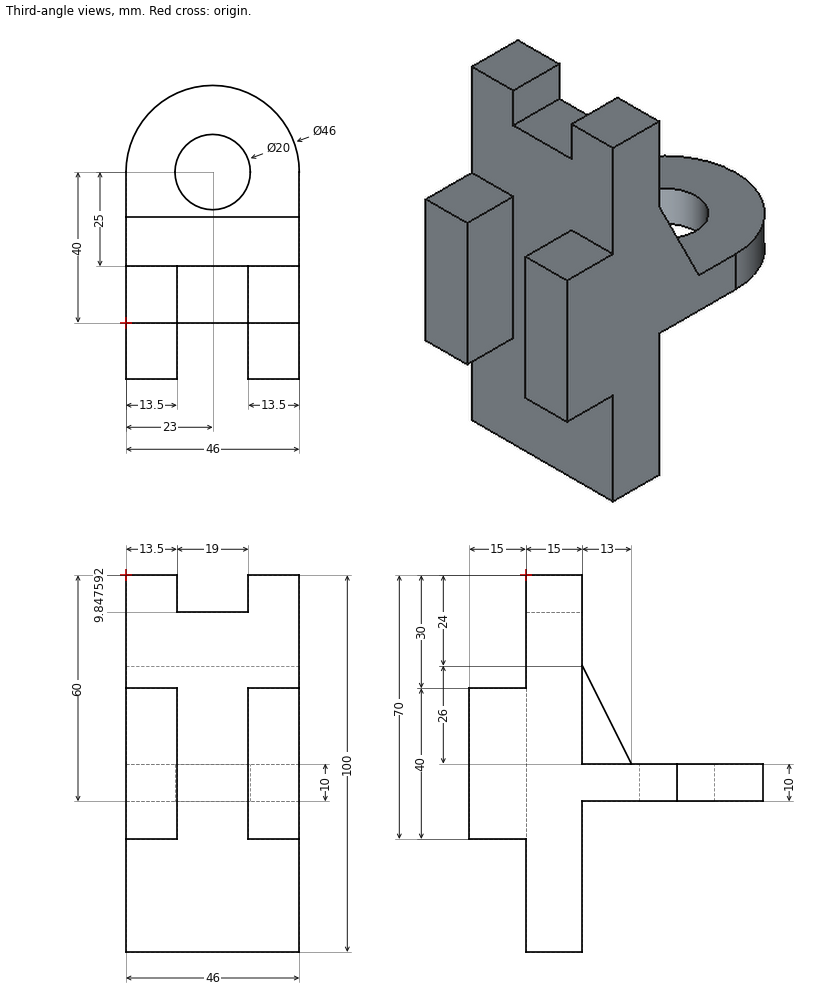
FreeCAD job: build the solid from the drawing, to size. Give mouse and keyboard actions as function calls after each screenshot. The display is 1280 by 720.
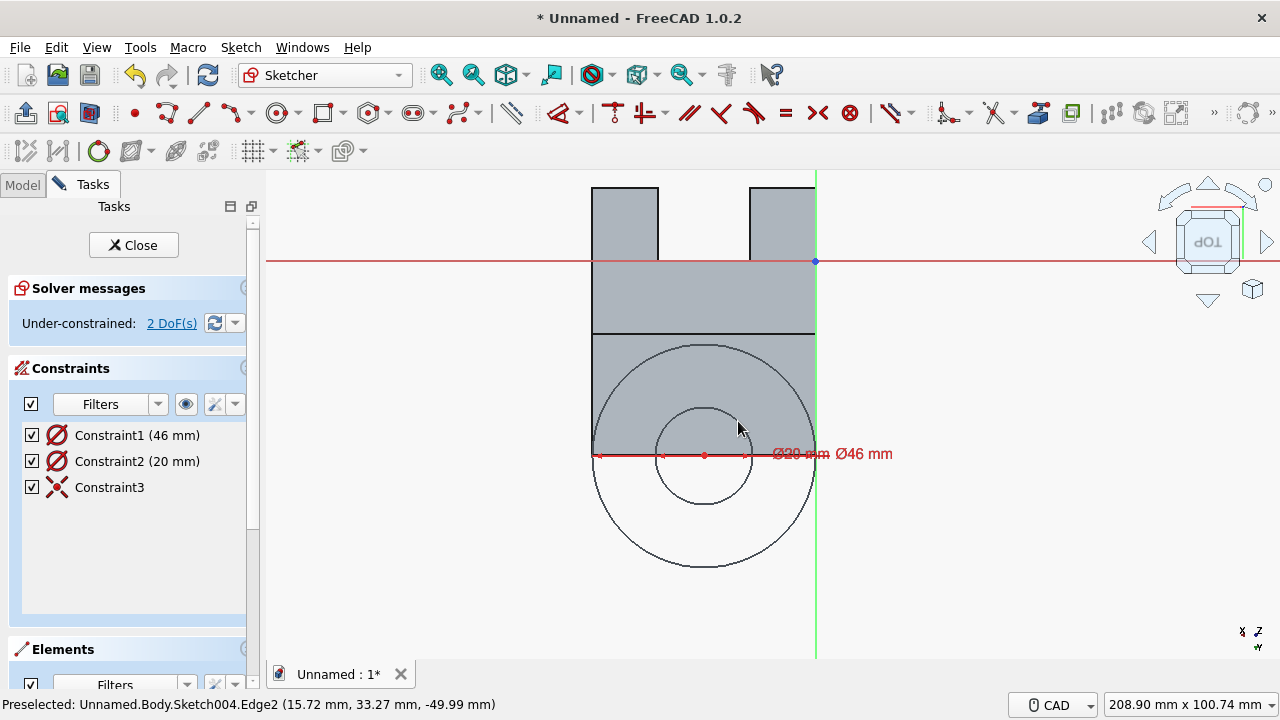
click(558, 114)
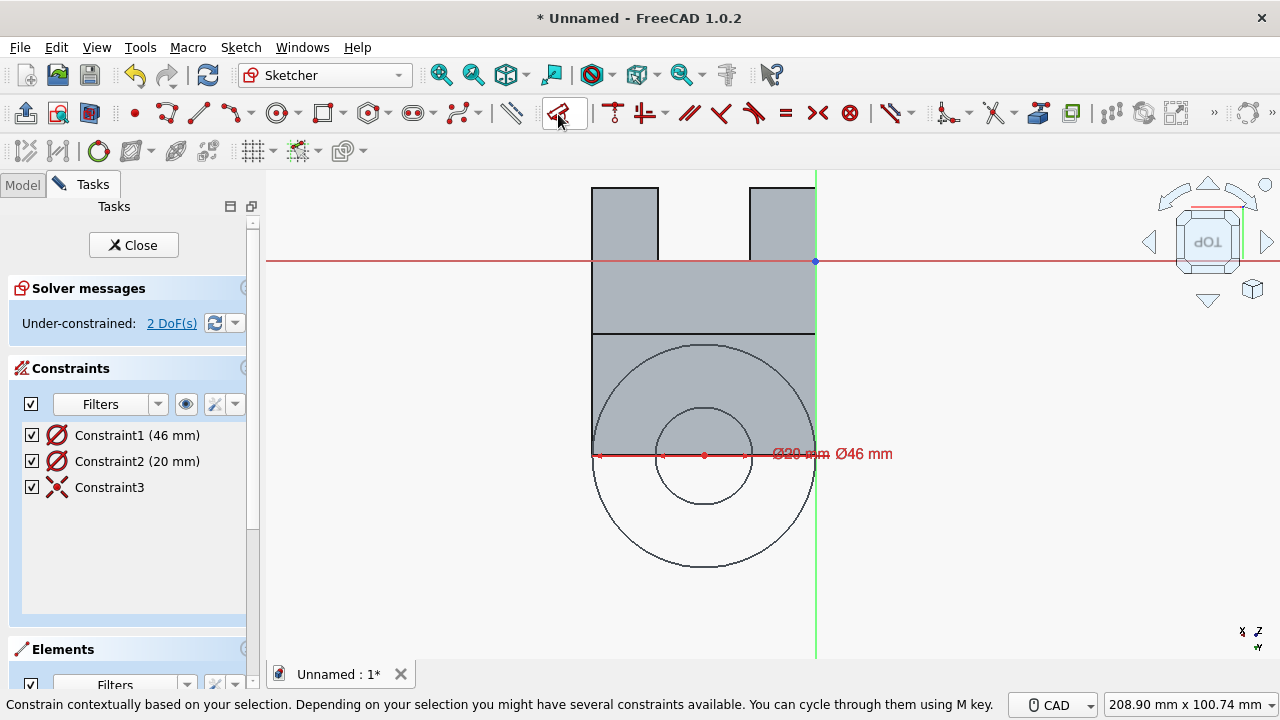
click(704, 456)
click(760, 227)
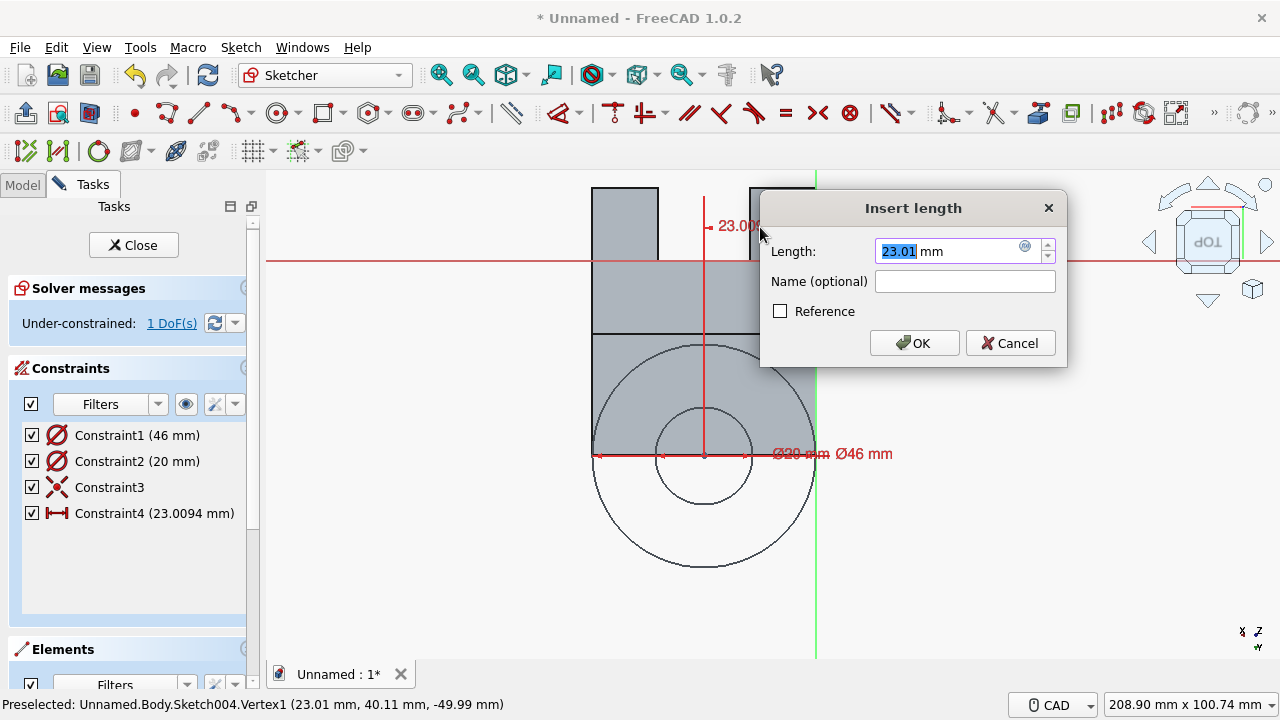
text(23)
key(Return)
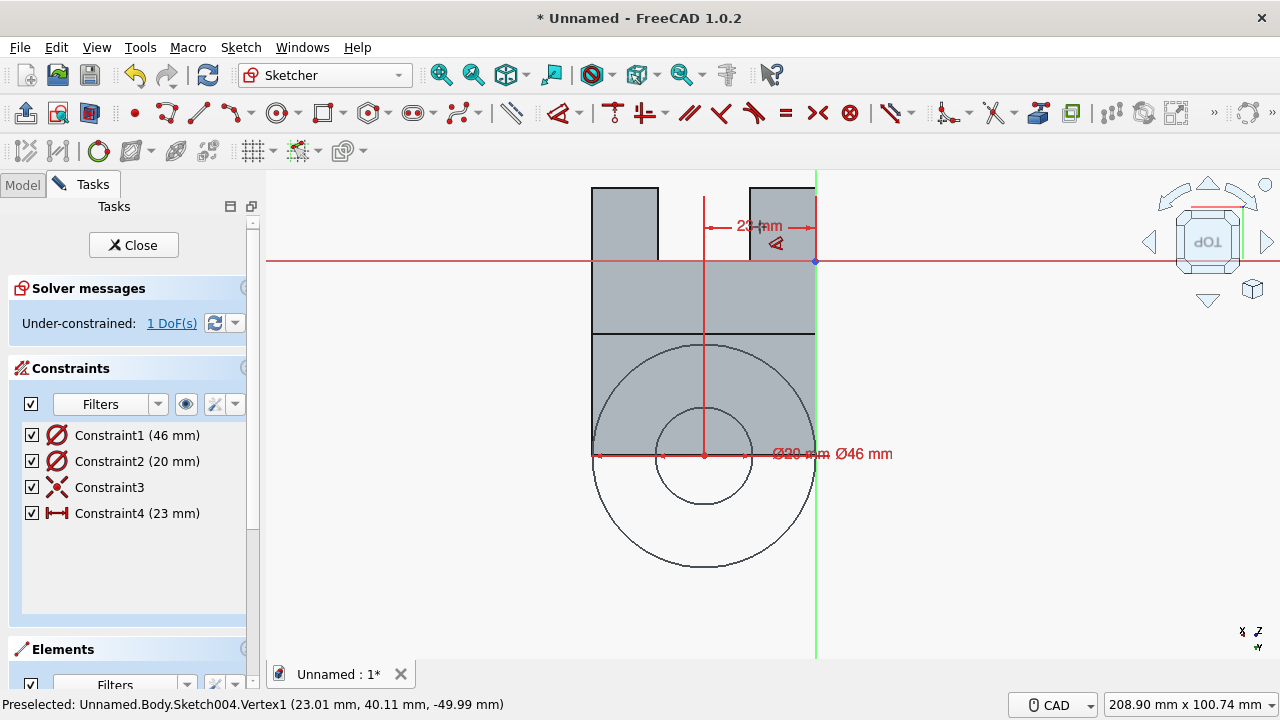
click(704, 456)
click(850, 359)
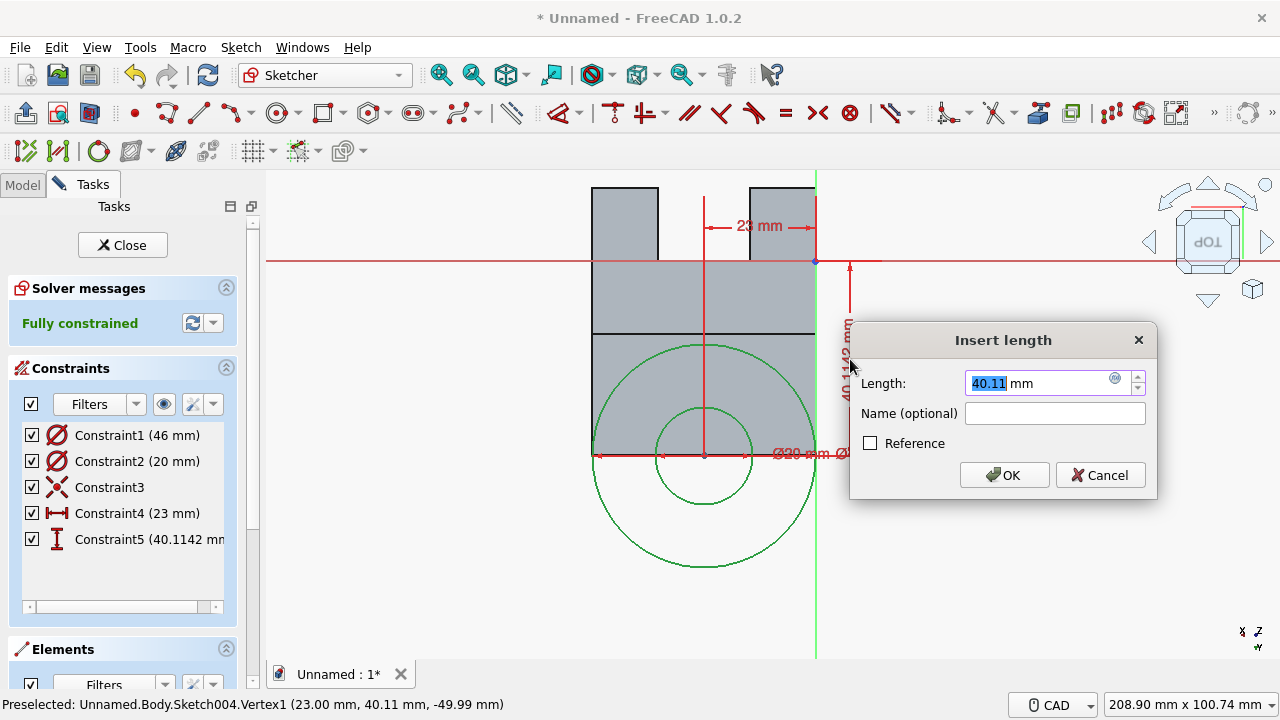
text(40)
key(Return)
key(Escape)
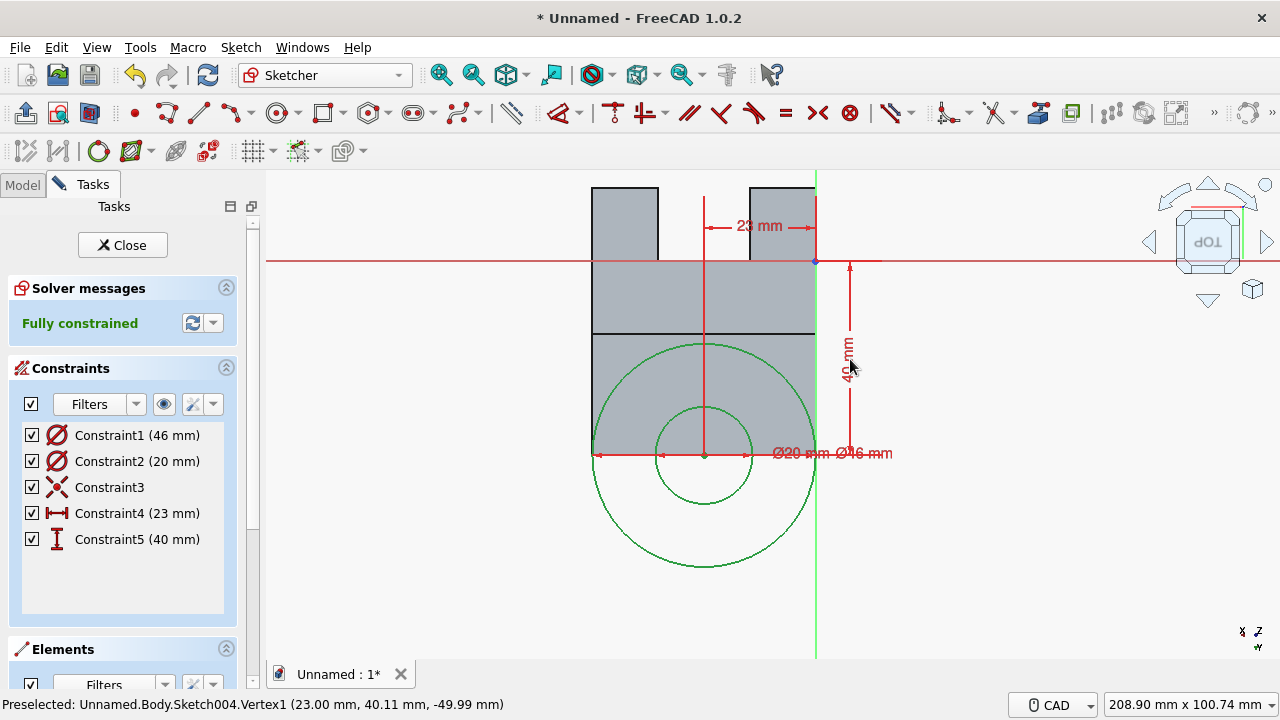
click(123, 245)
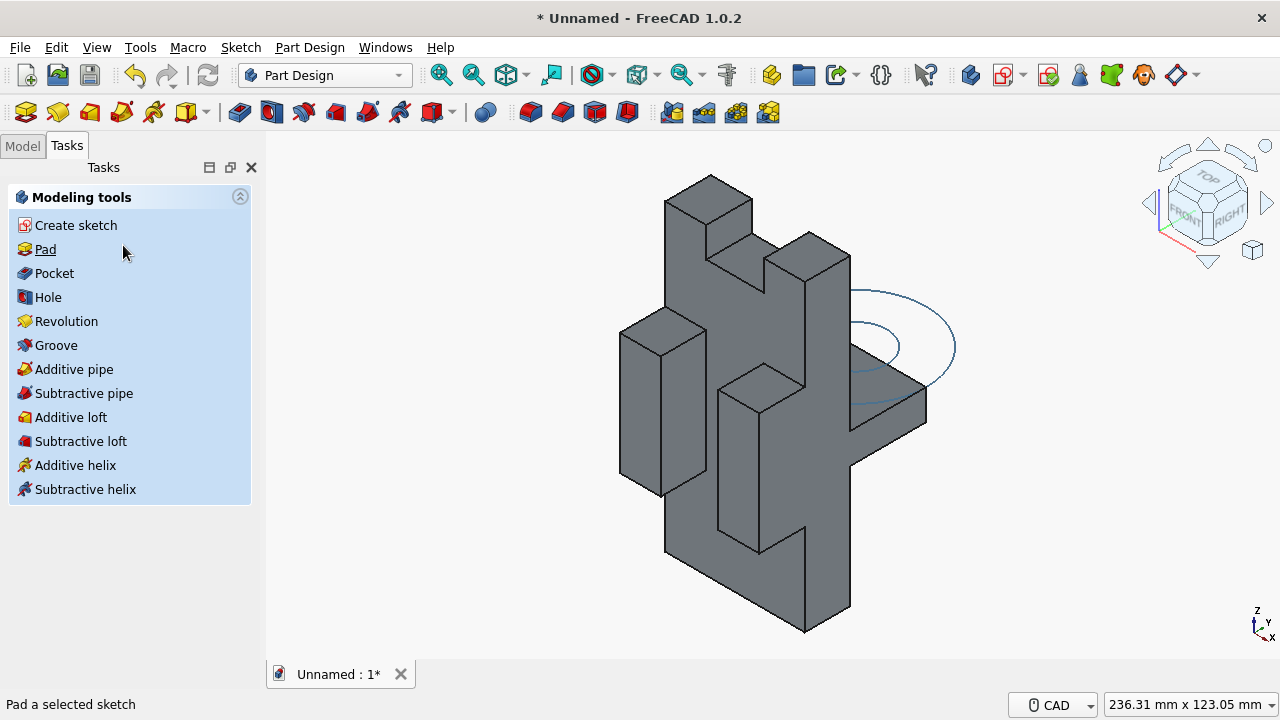
click(26, 112)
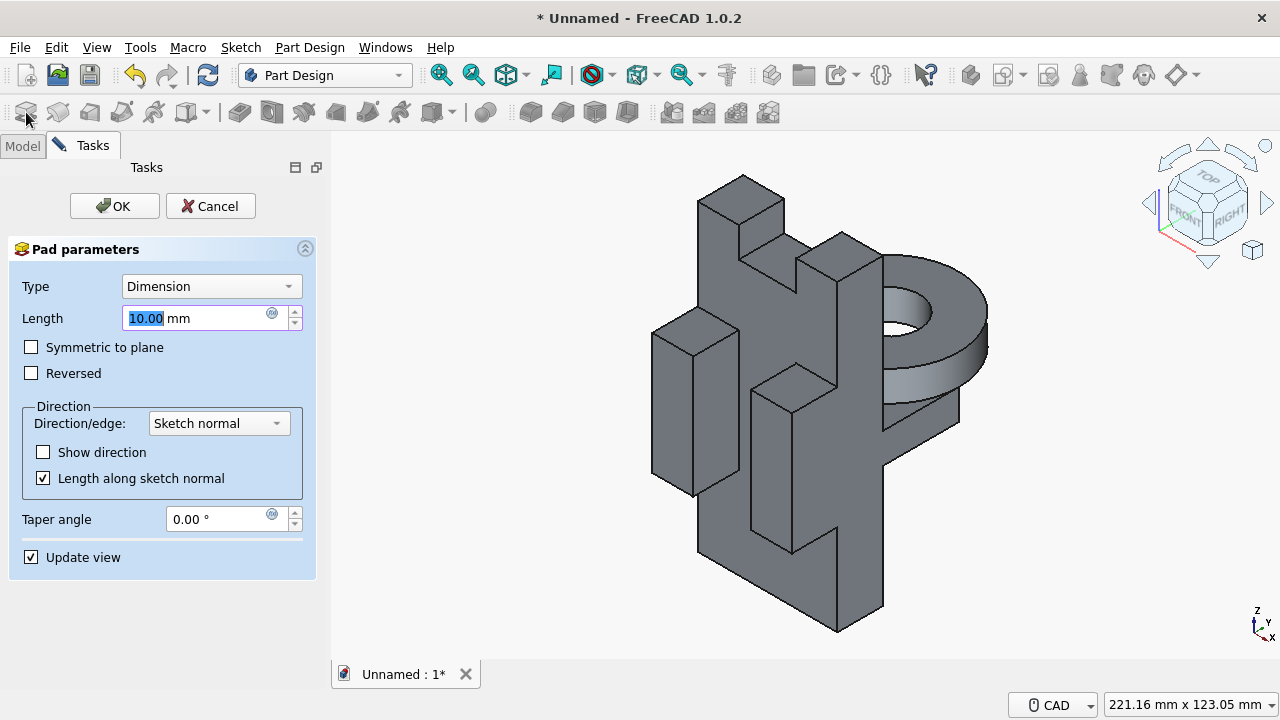
text(10)
key(Tab)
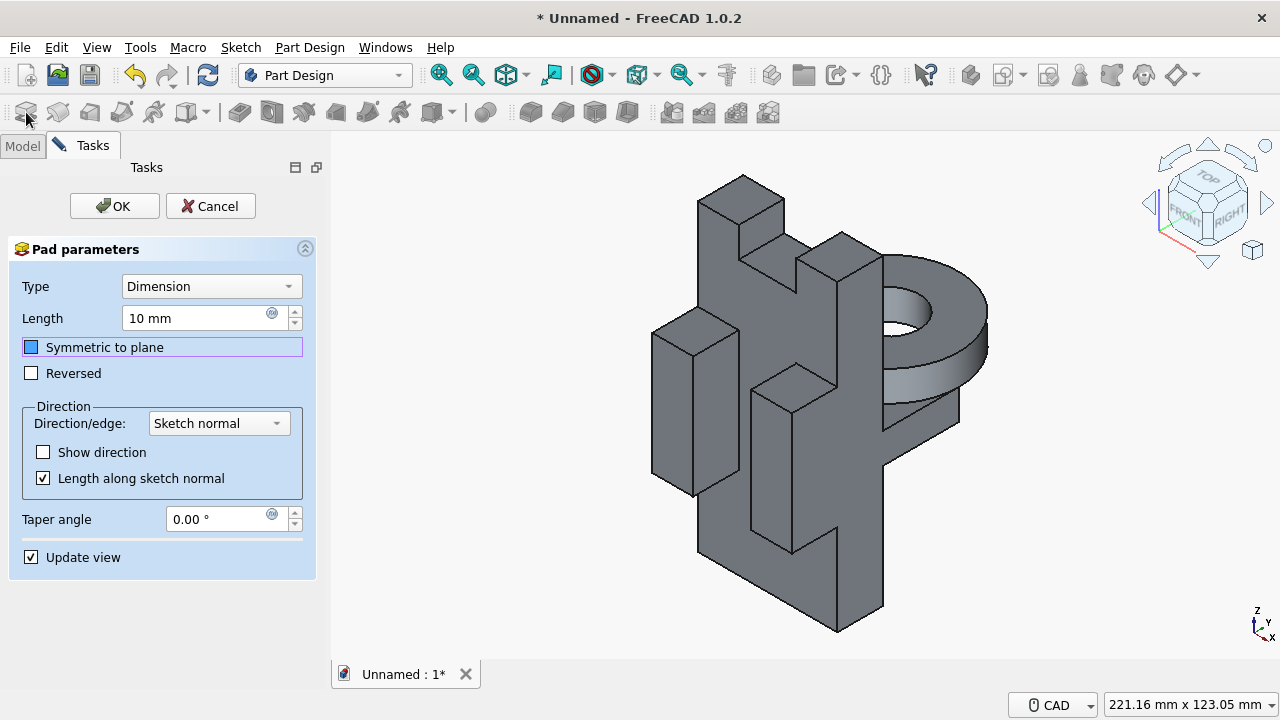
click(30, 373)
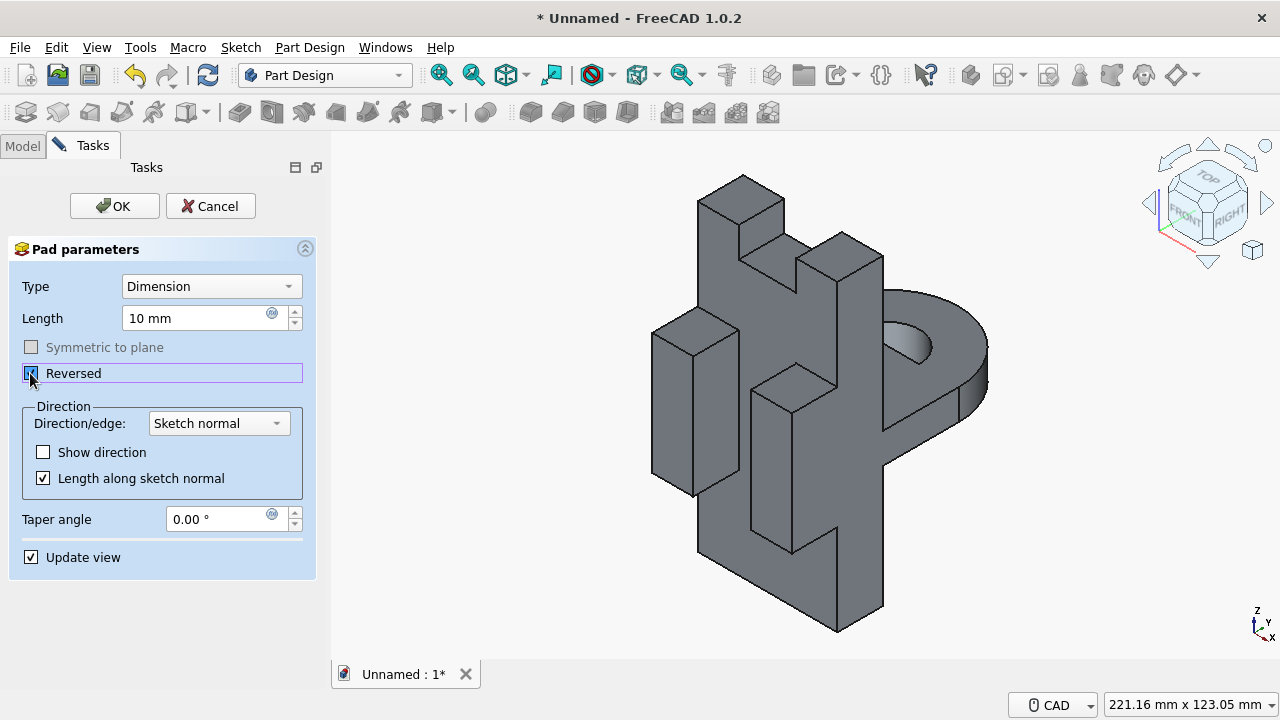
click(115, 206)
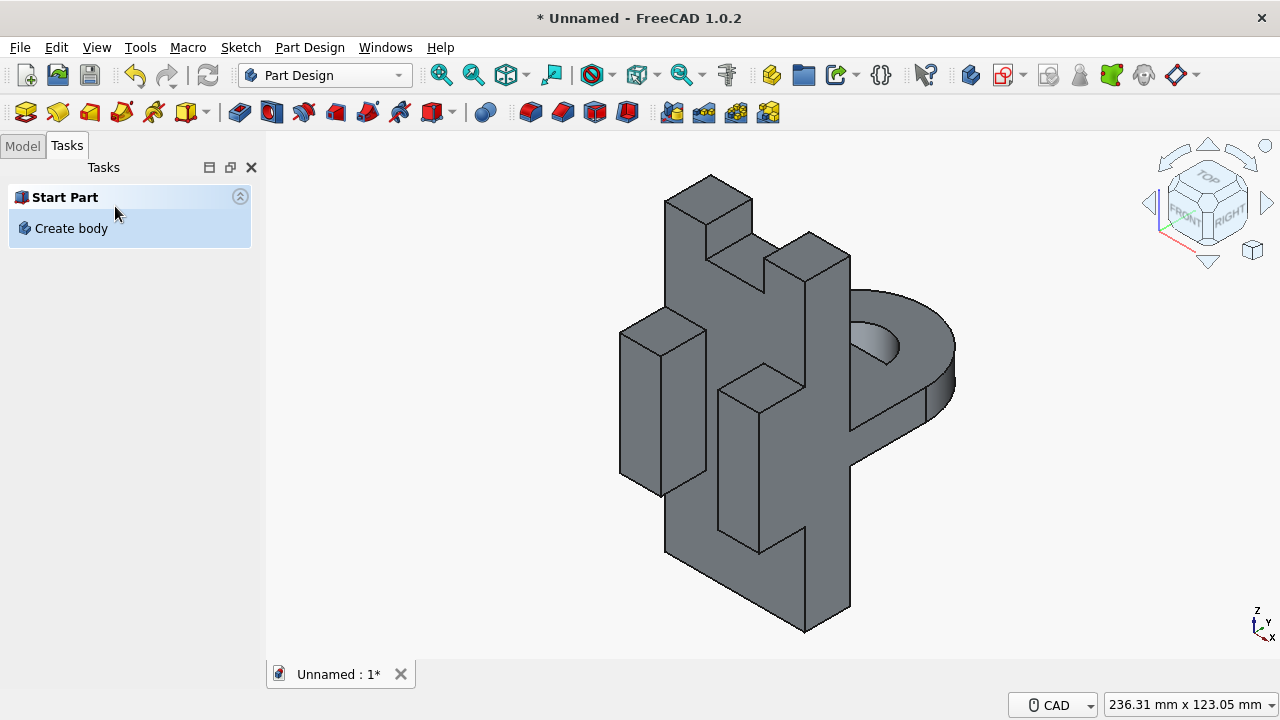
key(v)
key(f)